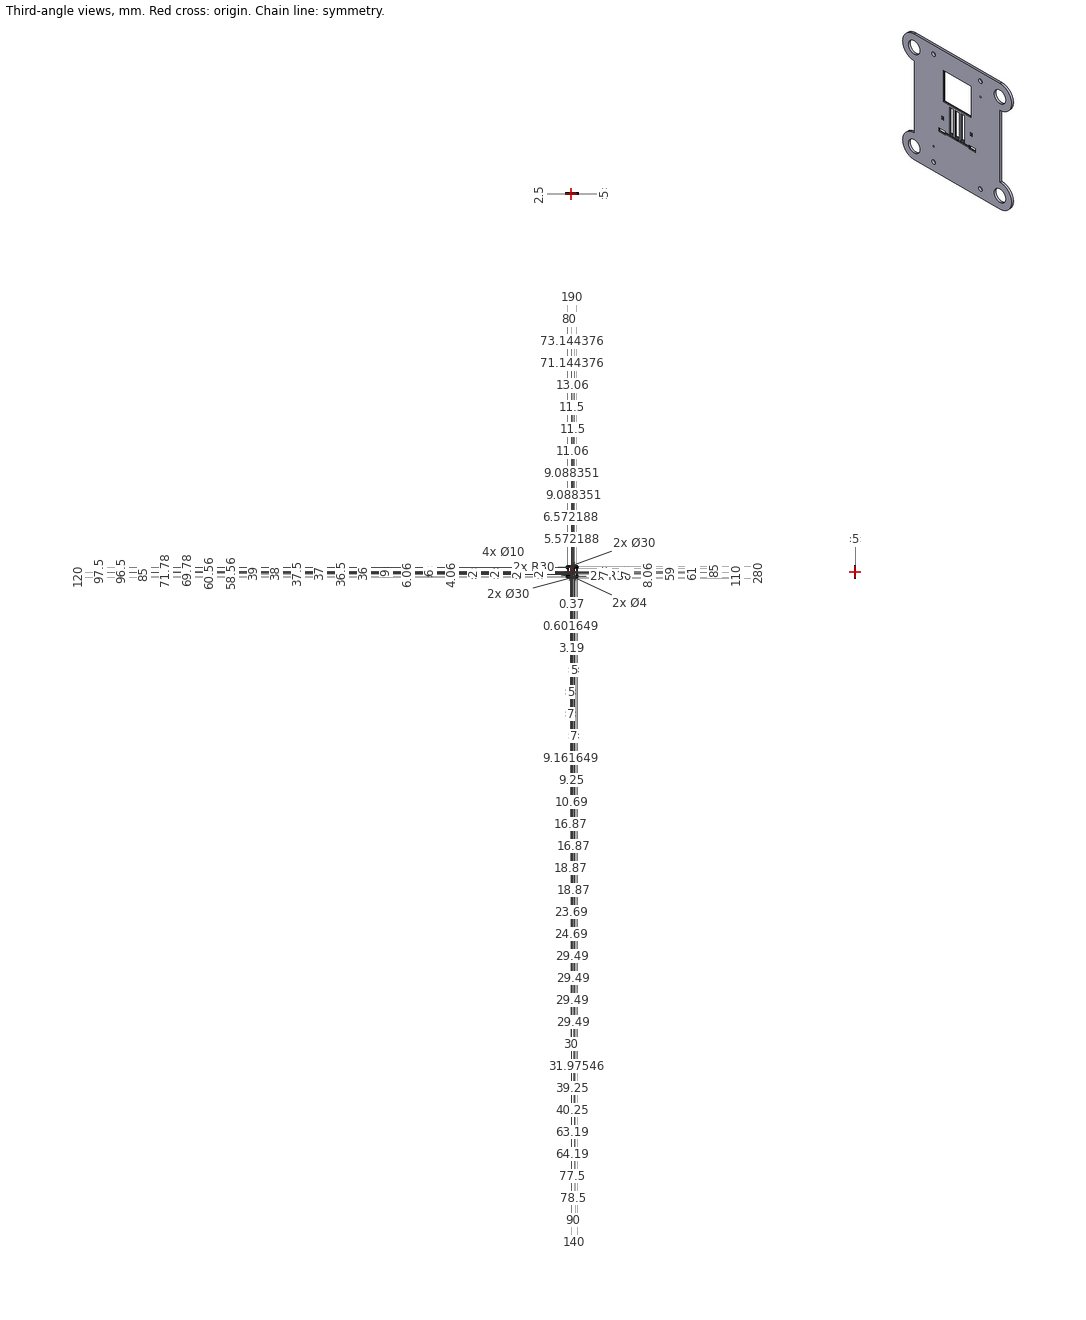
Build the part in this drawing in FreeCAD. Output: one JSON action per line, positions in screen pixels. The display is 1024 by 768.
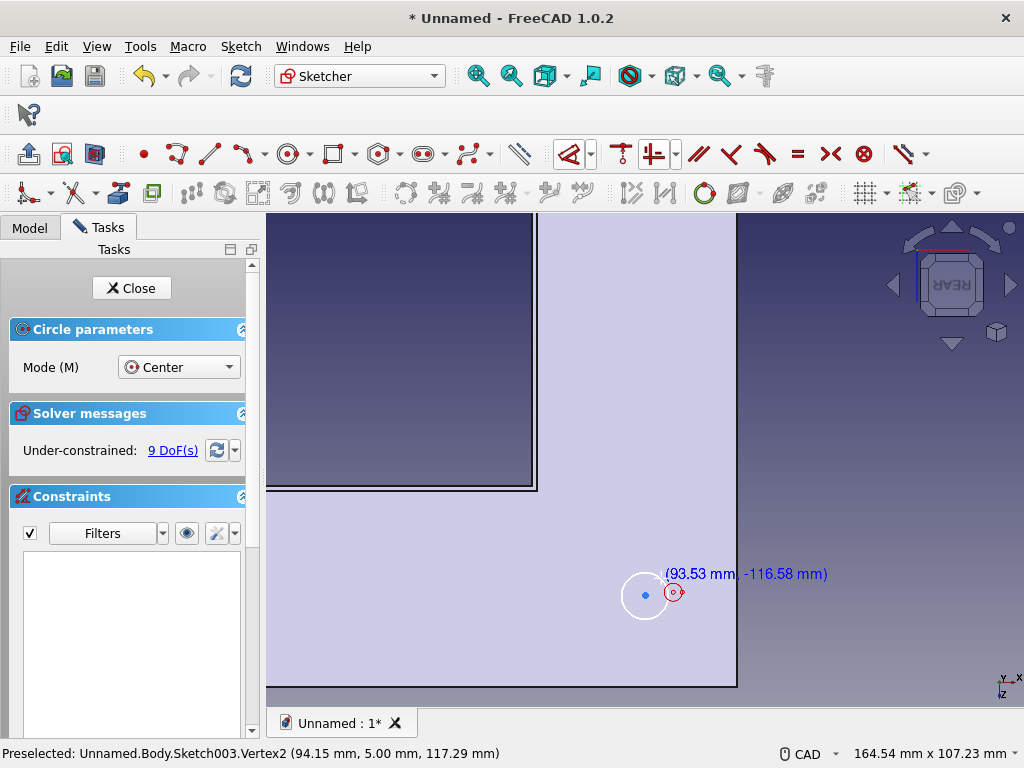
{"action": "scroll", "coordinate": [645, 597], "scroll_direction": "down", "scroll_amount": 7}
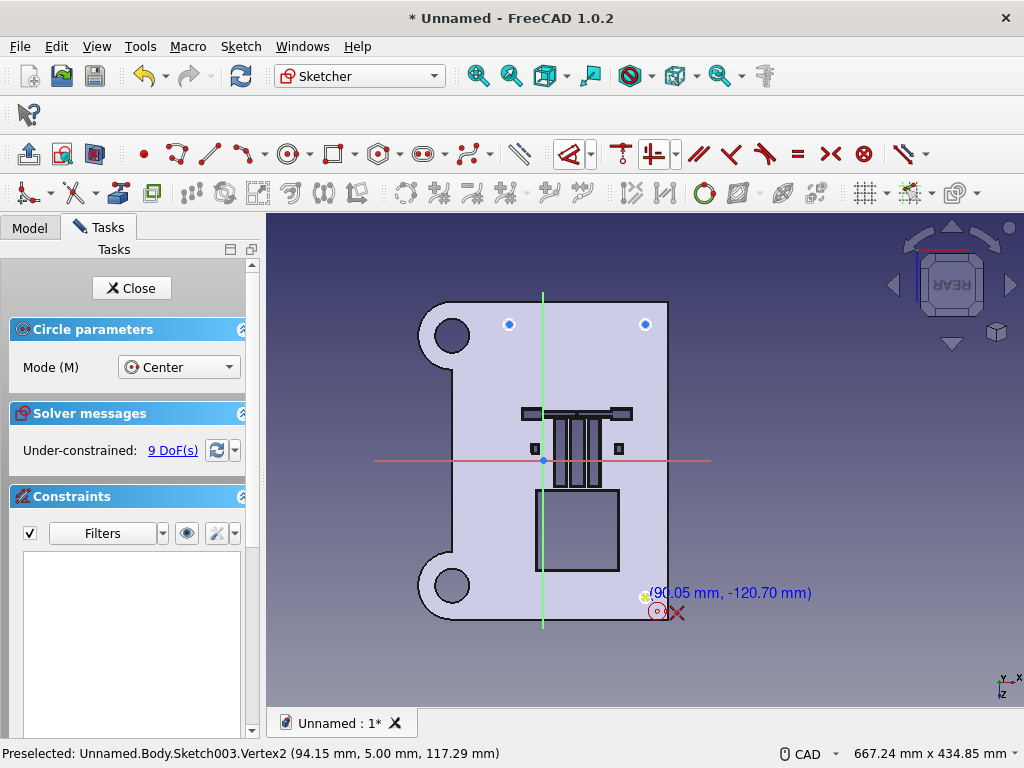
{"action": "scroll", "coordinate": [509, 597], "scroll_direction": "up", "scroll_amount": 7}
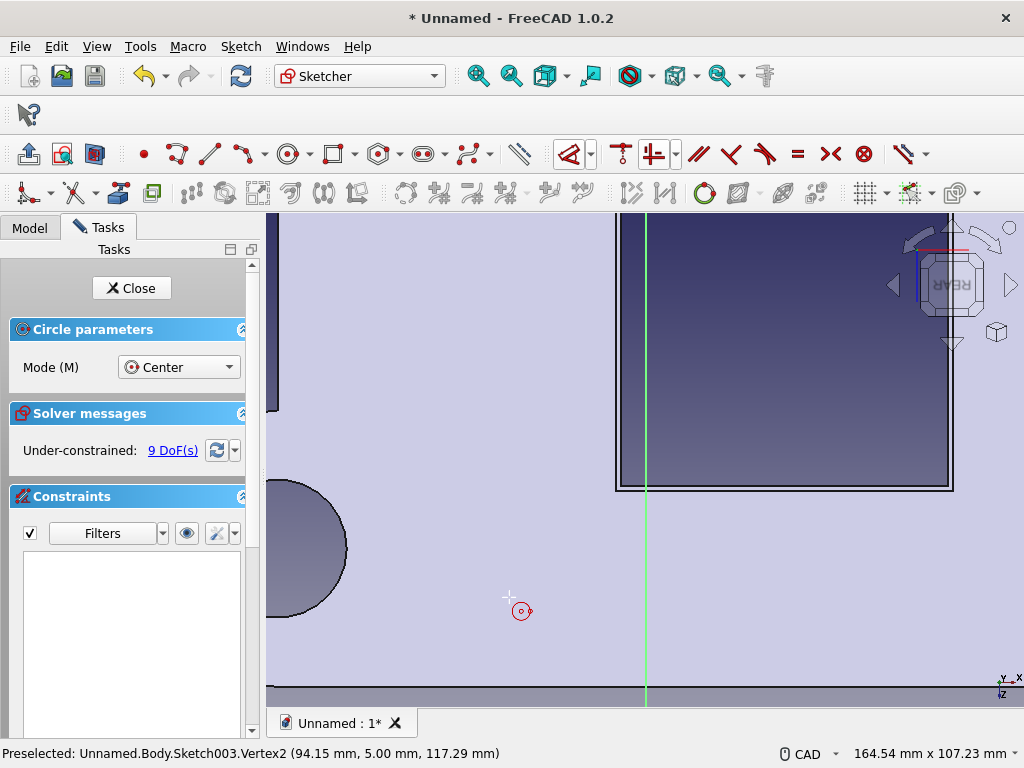
{"action": "left_click", "coordinate": [508, 595]}
{"action": "left_click", "coordinate": [524, 578]}
{"action": "key", "text": "Escape"}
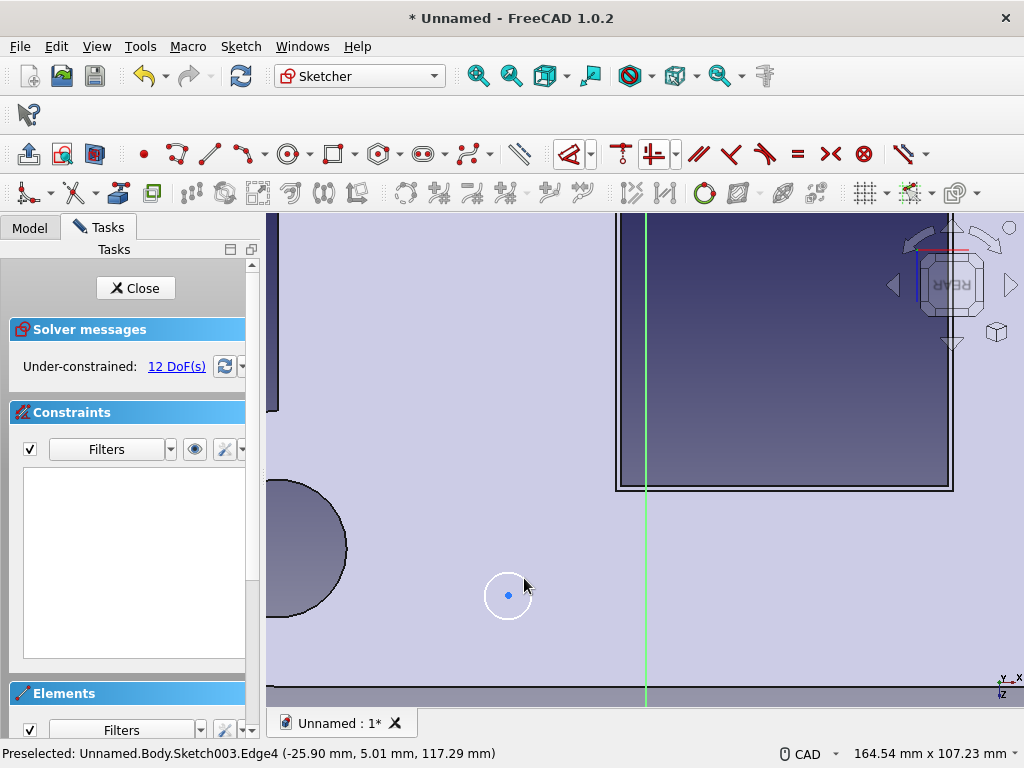
{"action": "scroll", "coordinate": [508, 597], "scroll_direction": "down", "scroll_amount": 7}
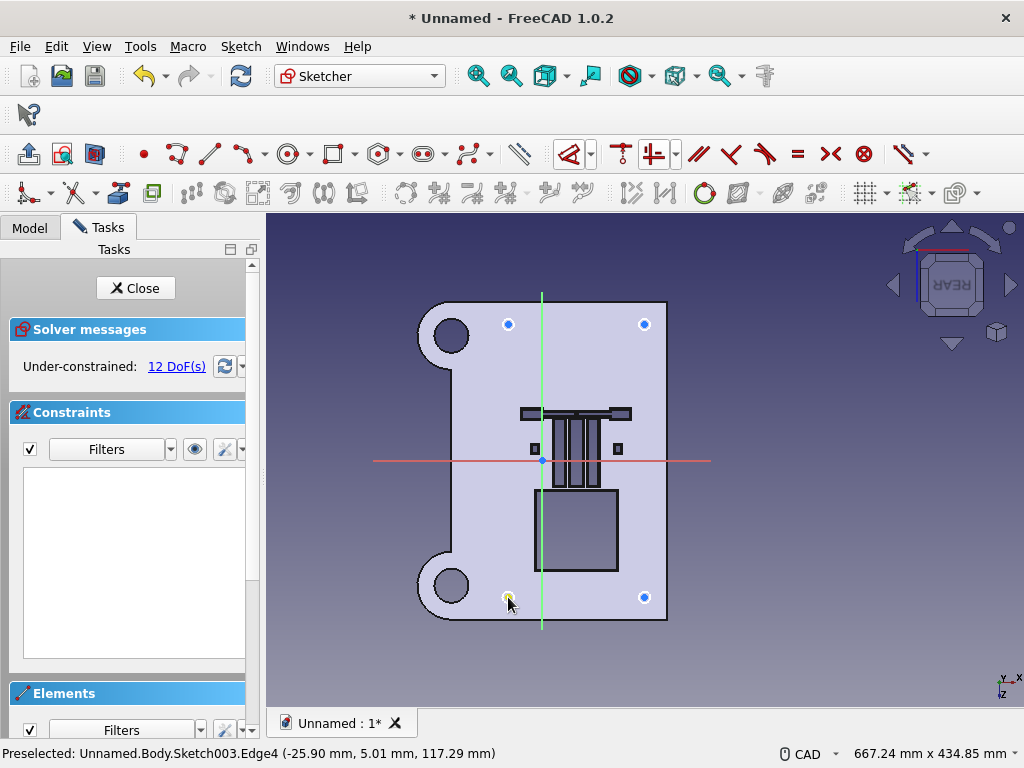
{"action": "scroll", "coordinate": [512, 321], "scroll_direction": "up", "scroll_amount": 5}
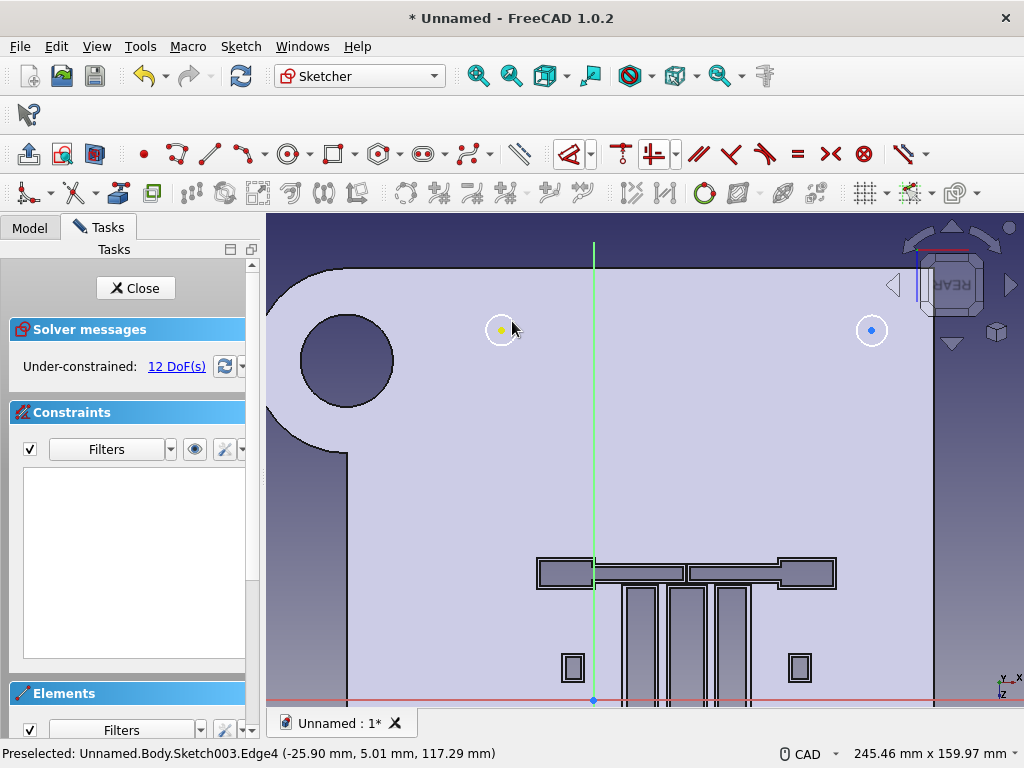
{"action": "left_click", "coordinate": [512, 320]}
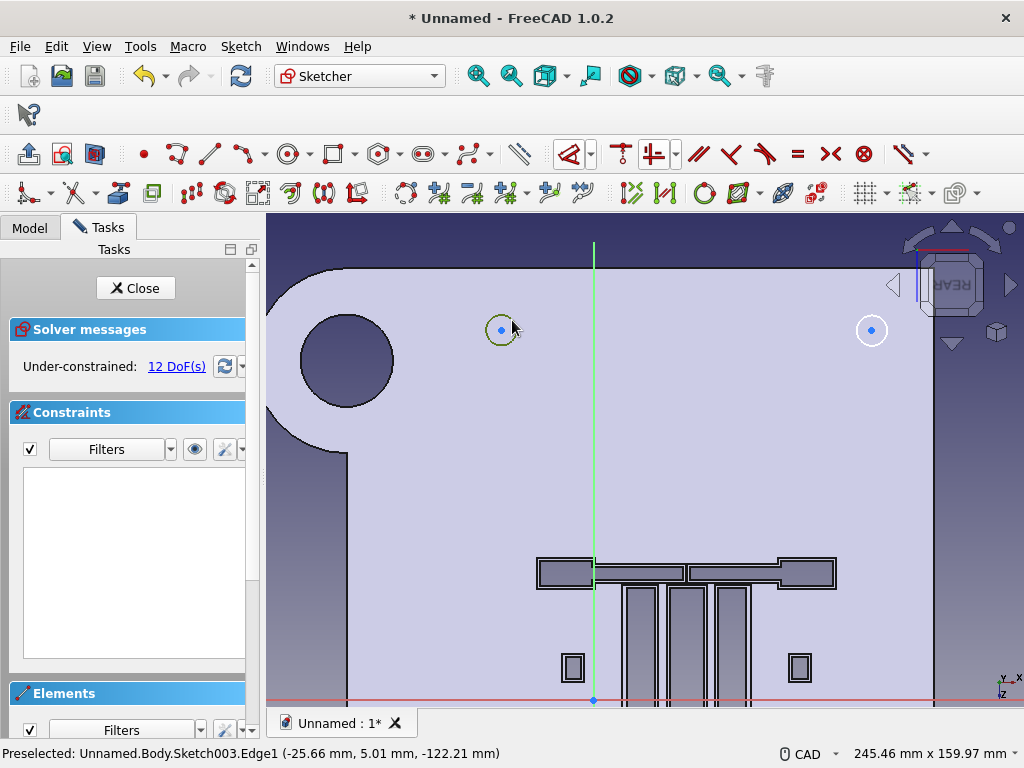
{"action": "left_click", "coordinate": [857, 330]}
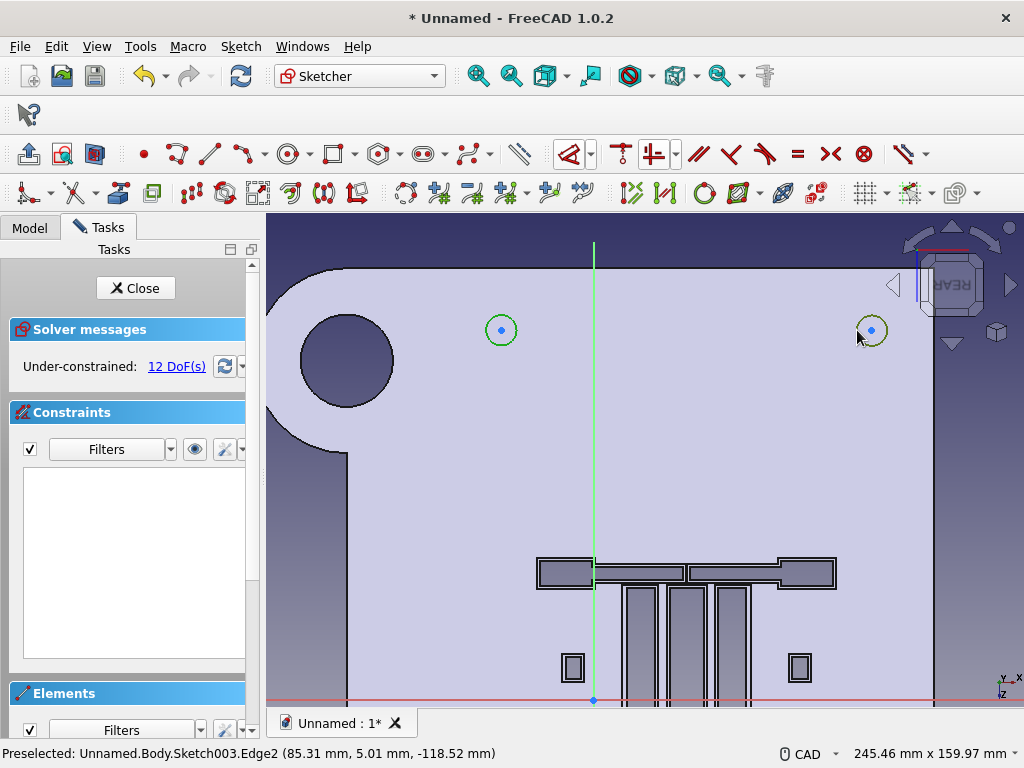
{"action": "scroll", "coordinate": [512, 320], "scroll_direction": "down", "scroll_amount": 5}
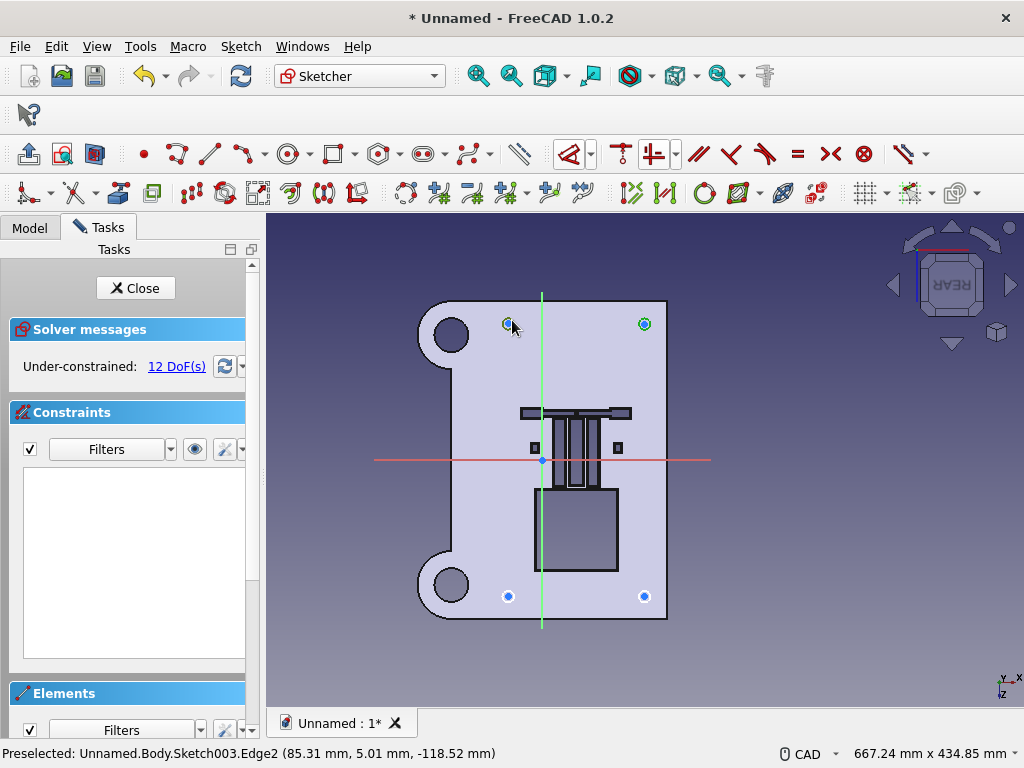
{"action": "scroll", "coordinate": [649, 593], "scroll_direction": "up", "scroll_amount": 5}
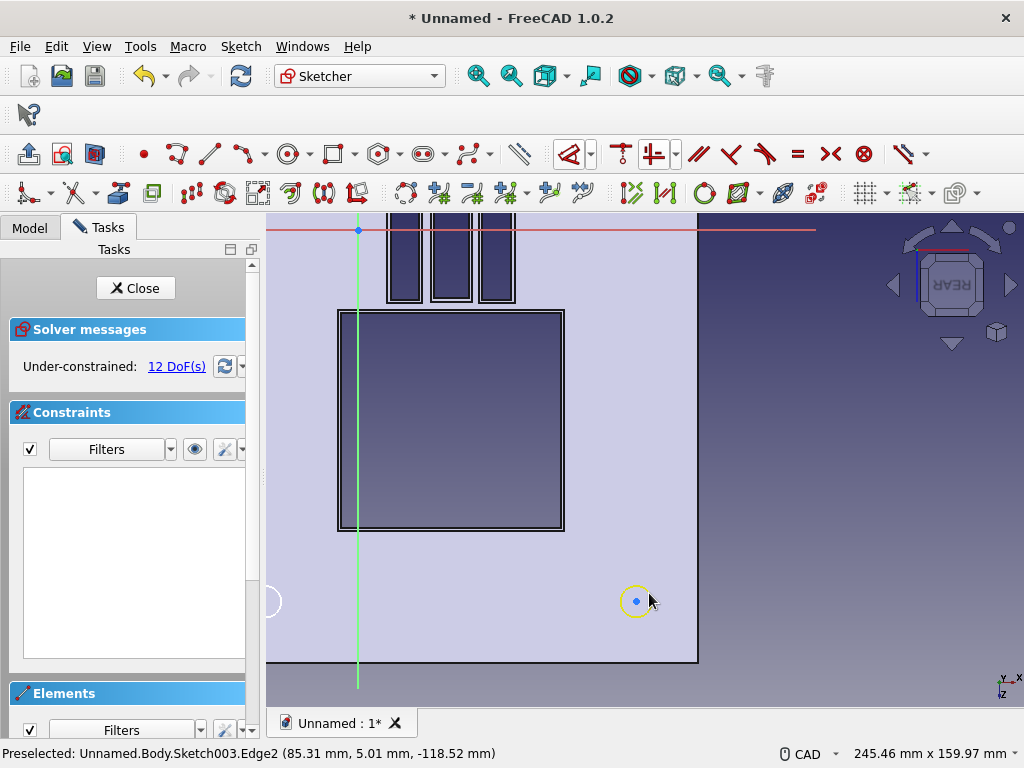
{"action": "left_click", "coordinate": [647, 591]}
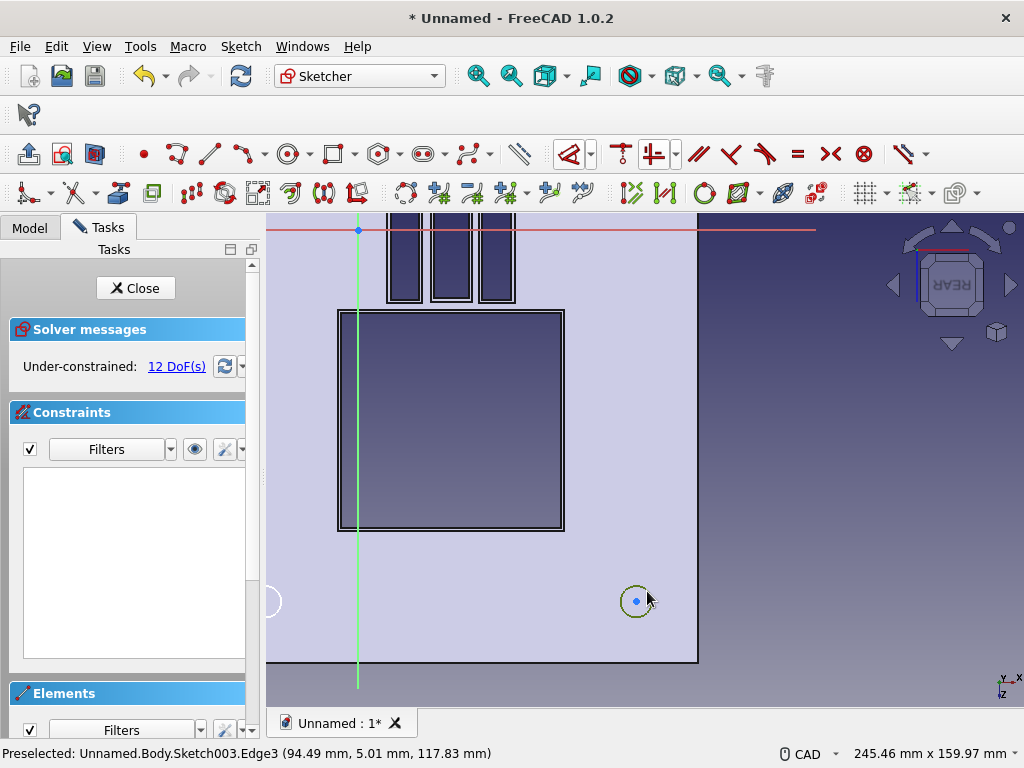
{"action": "scroll", "coordinate": [650, 594], "scroll_direction": "down", "scroll_amount": 5}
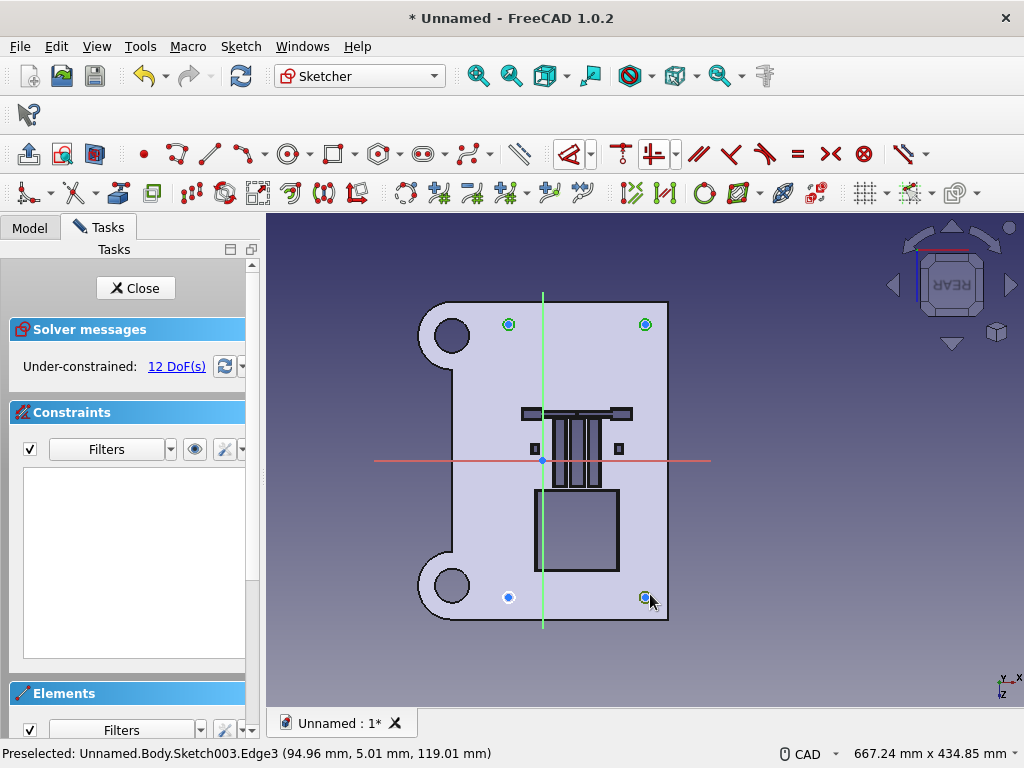
{"action": "scroll", "coordinate": [513, 593], "scroll_direction": "up", "scroll_amount": 5}